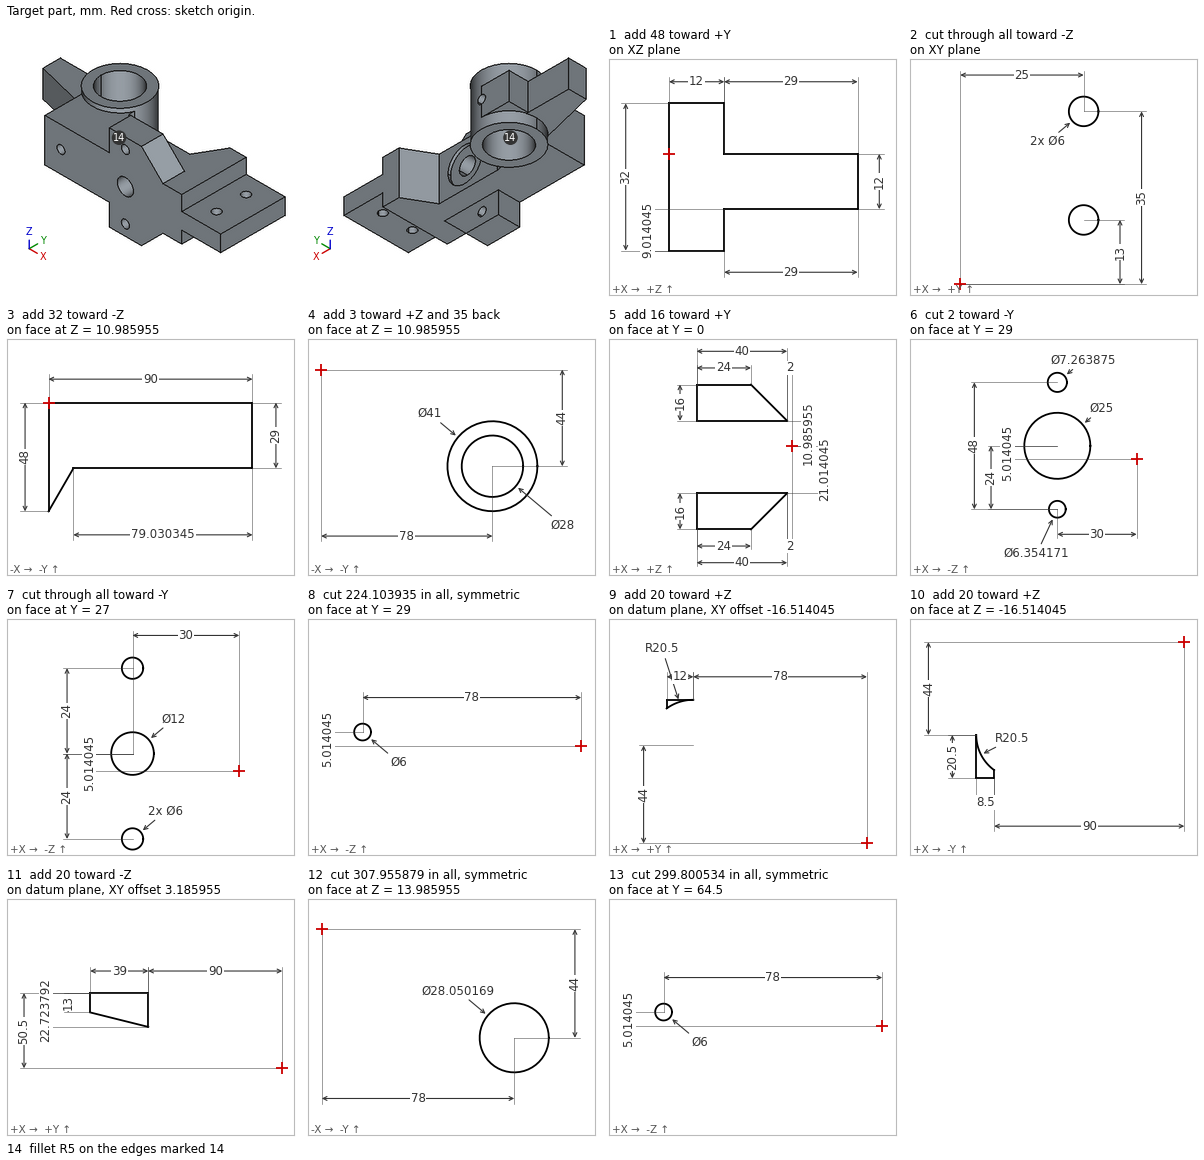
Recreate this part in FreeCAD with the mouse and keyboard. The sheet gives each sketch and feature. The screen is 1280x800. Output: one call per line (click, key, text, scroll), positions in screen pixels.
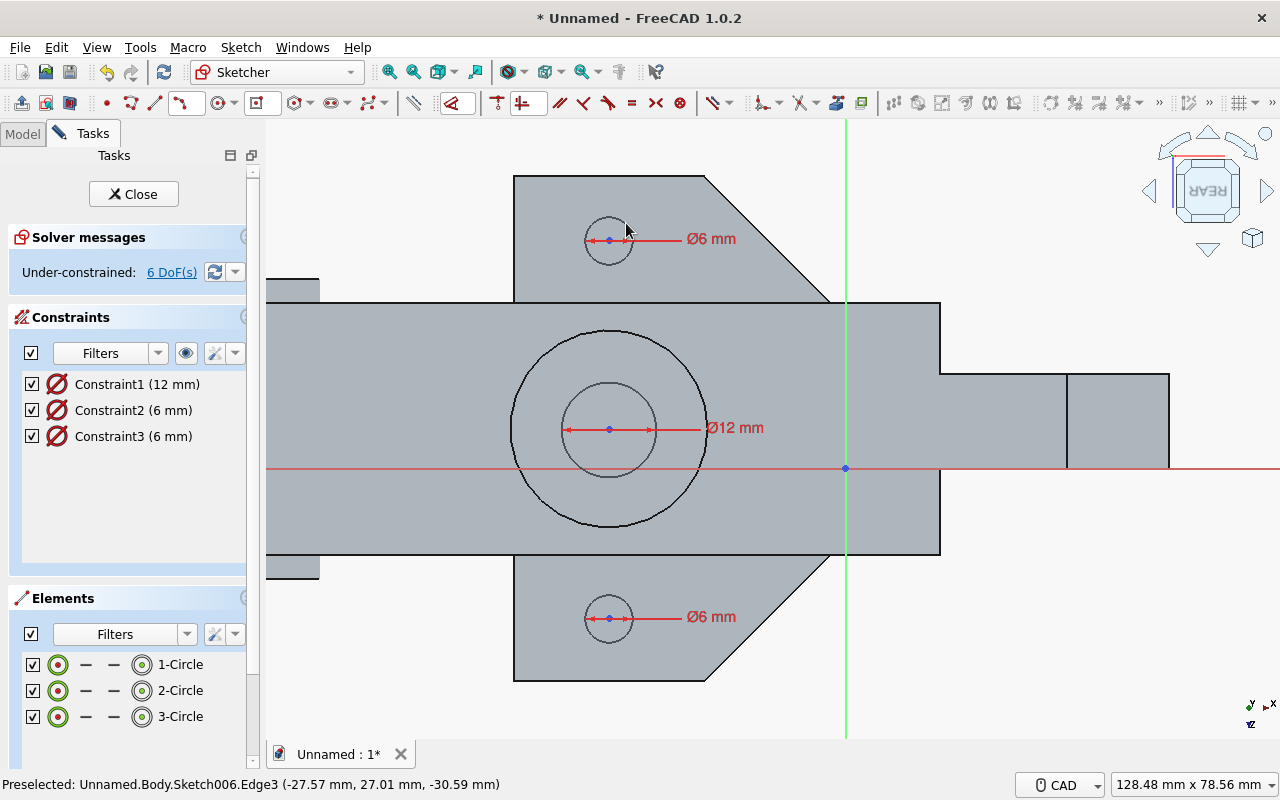
click(609, 430)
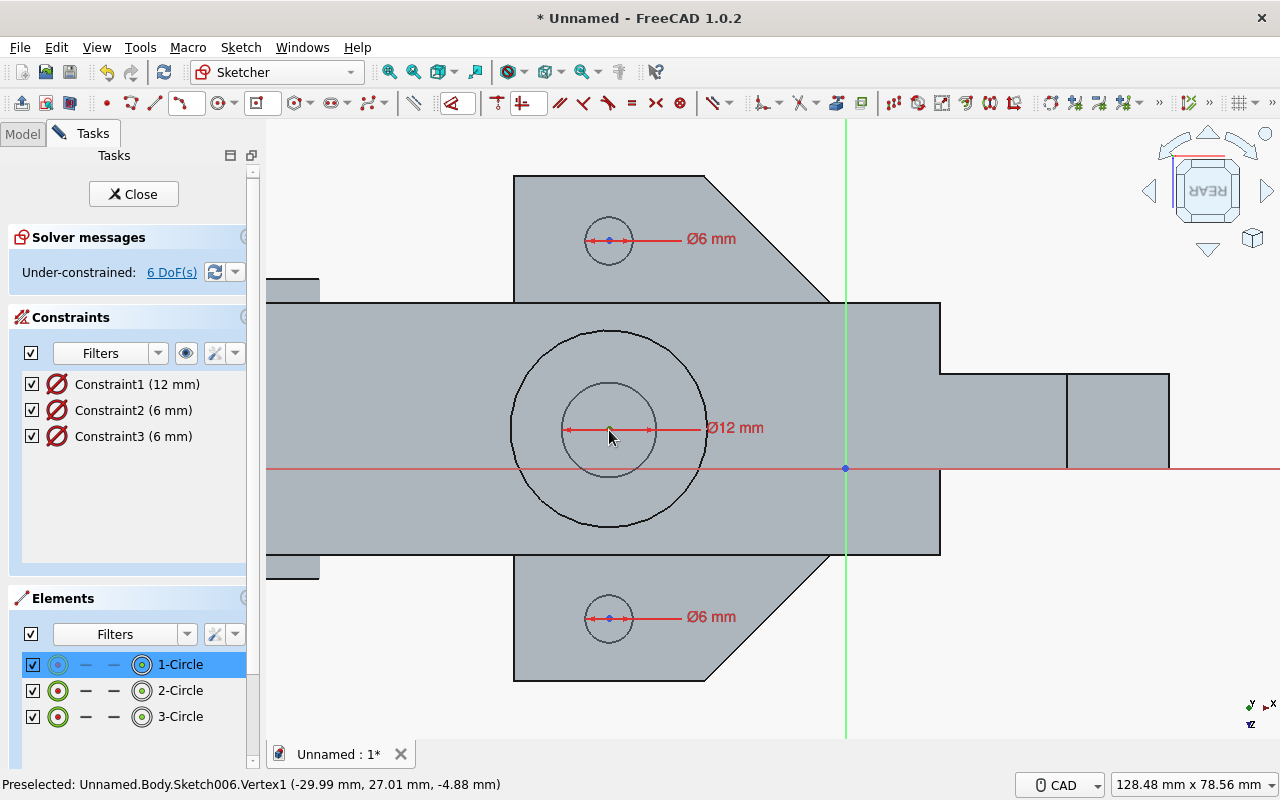
click(609, 619)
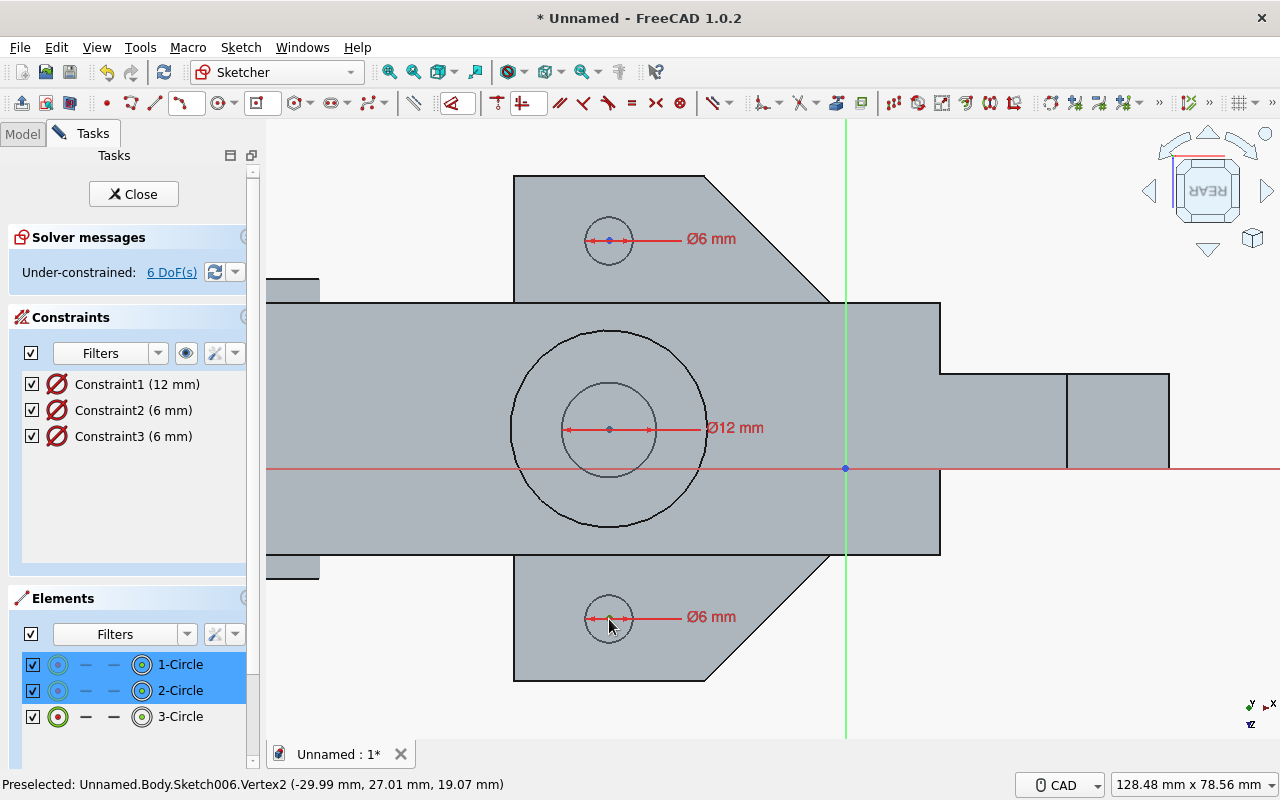
key(v)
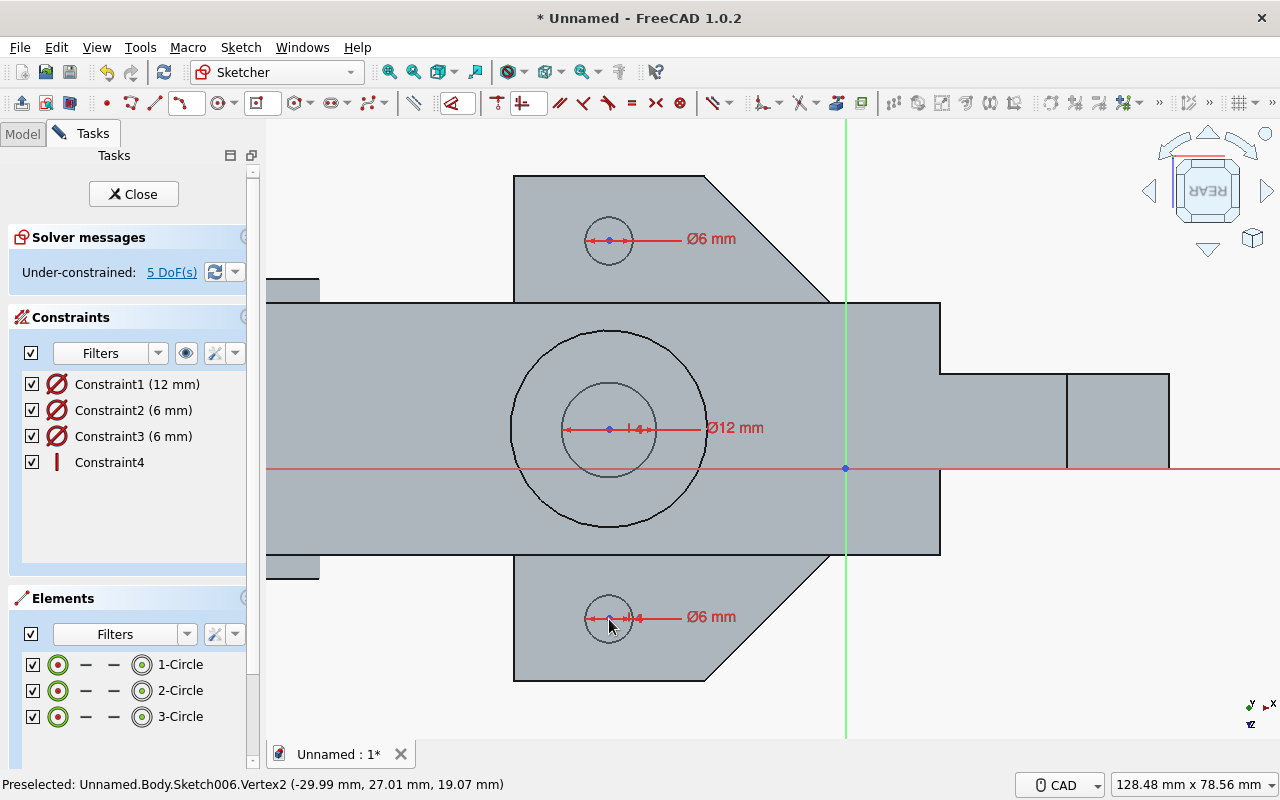
click(609, 430)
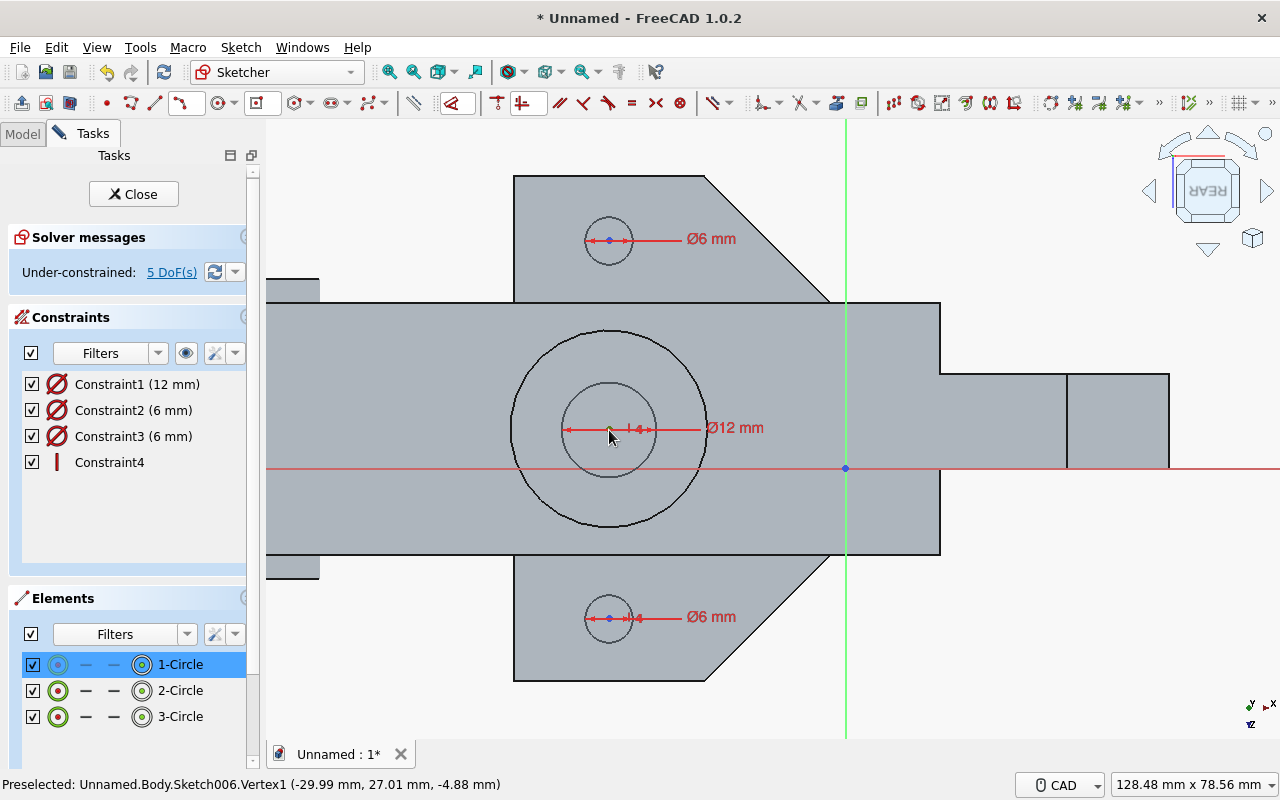
click(609, 241)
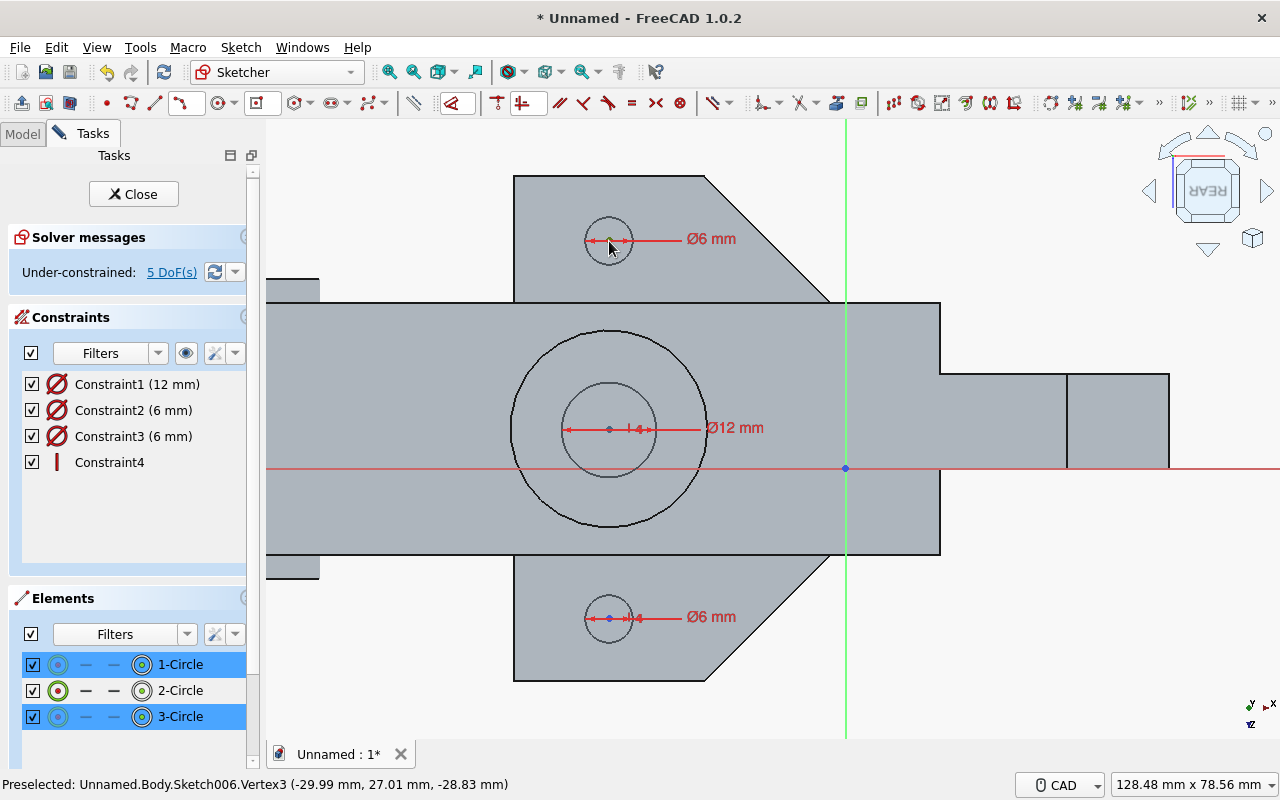
key(v)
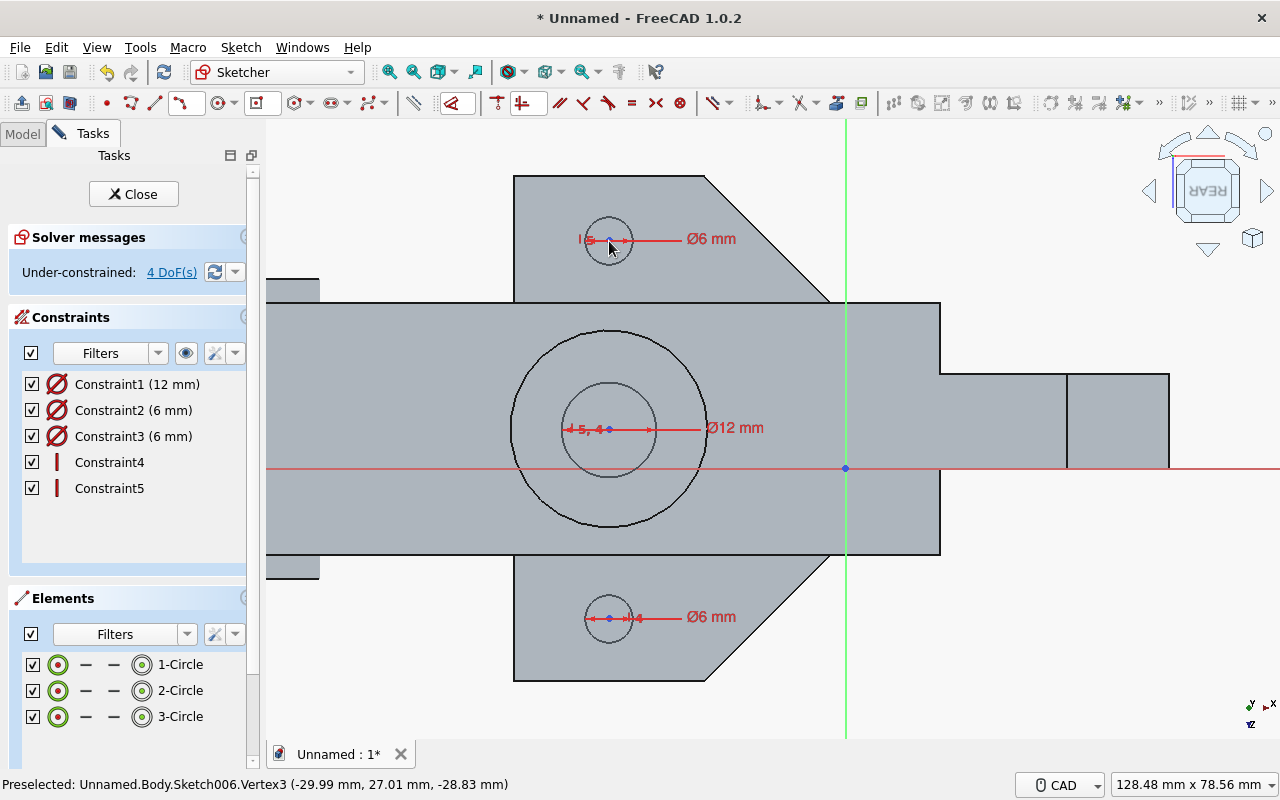
click(609, 430)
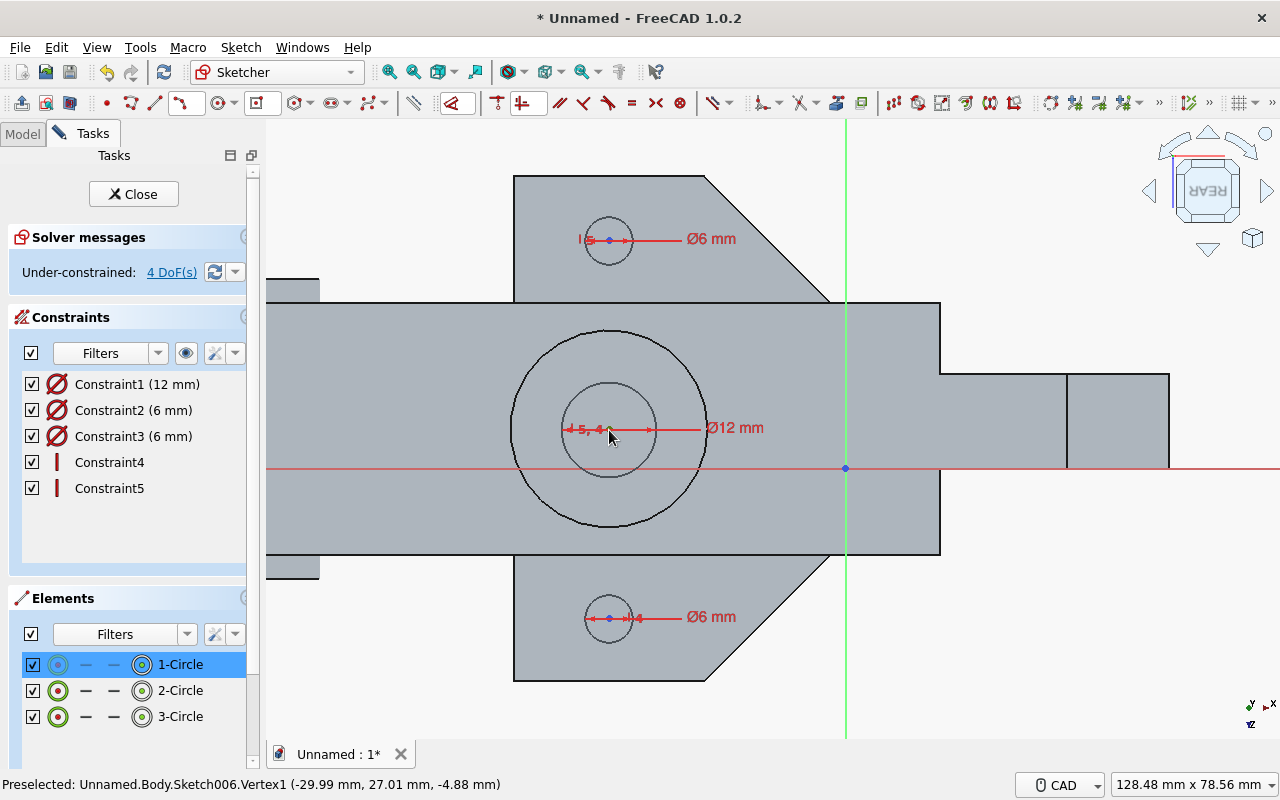
key(l)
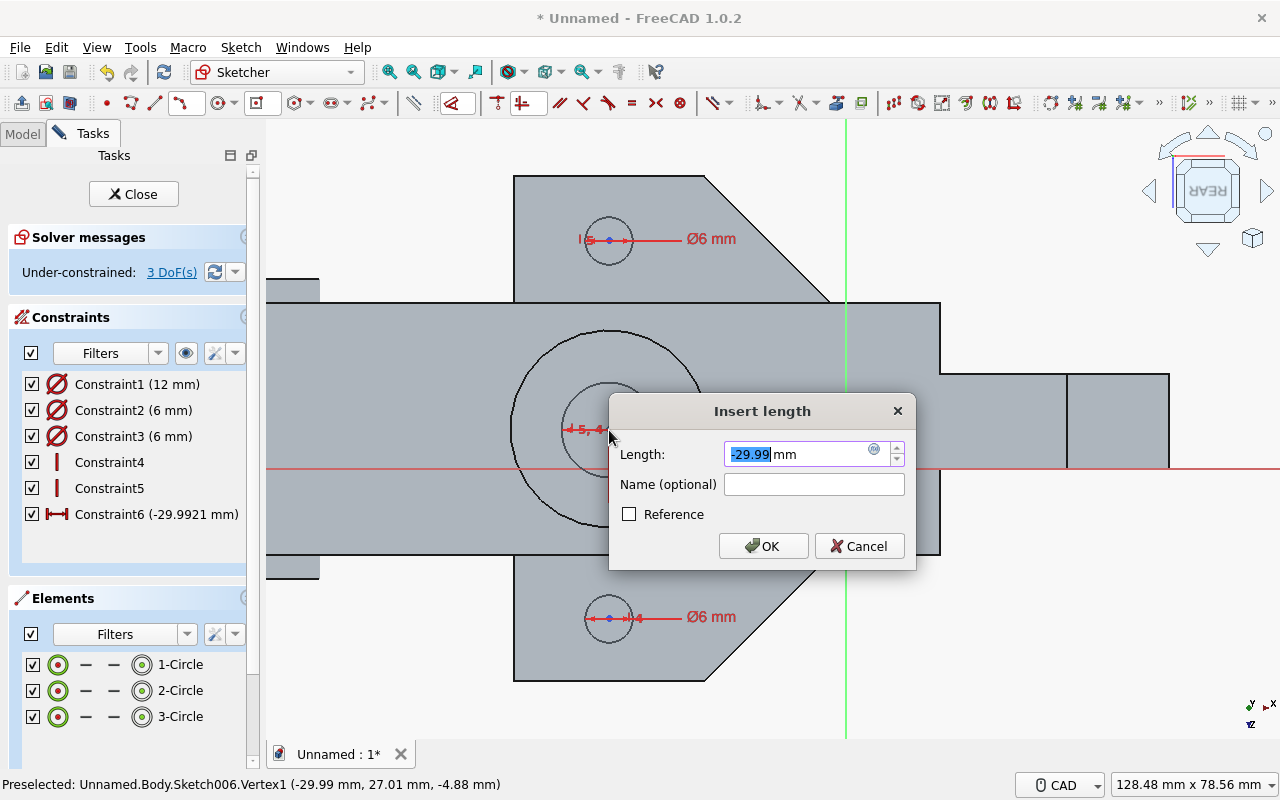
text(-30)
key(Return)